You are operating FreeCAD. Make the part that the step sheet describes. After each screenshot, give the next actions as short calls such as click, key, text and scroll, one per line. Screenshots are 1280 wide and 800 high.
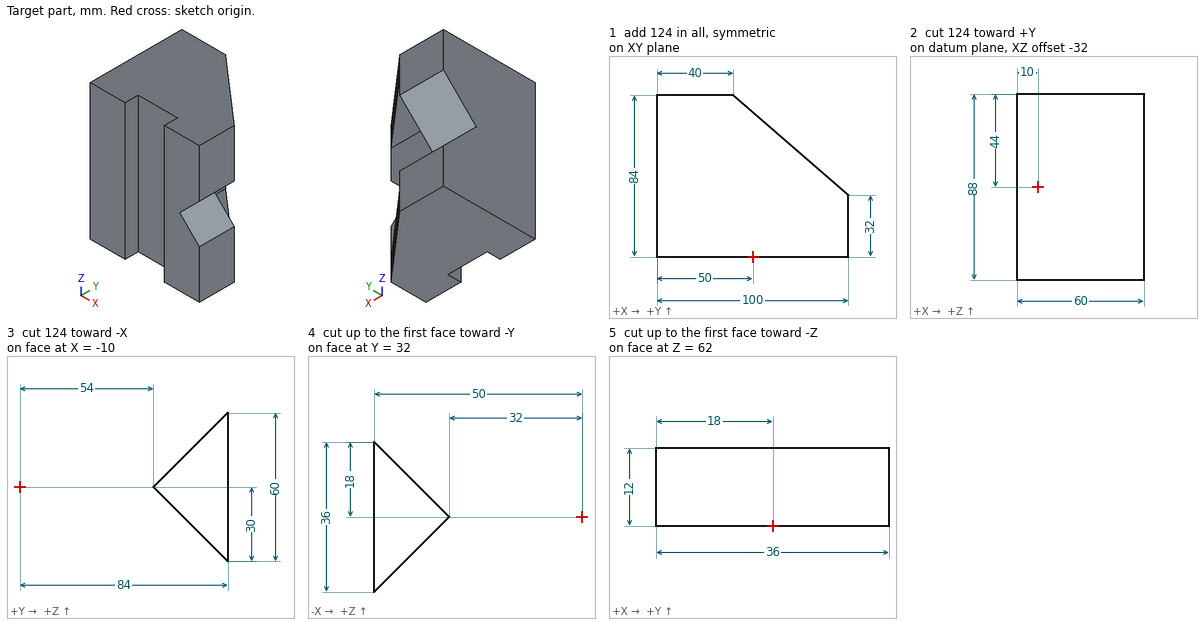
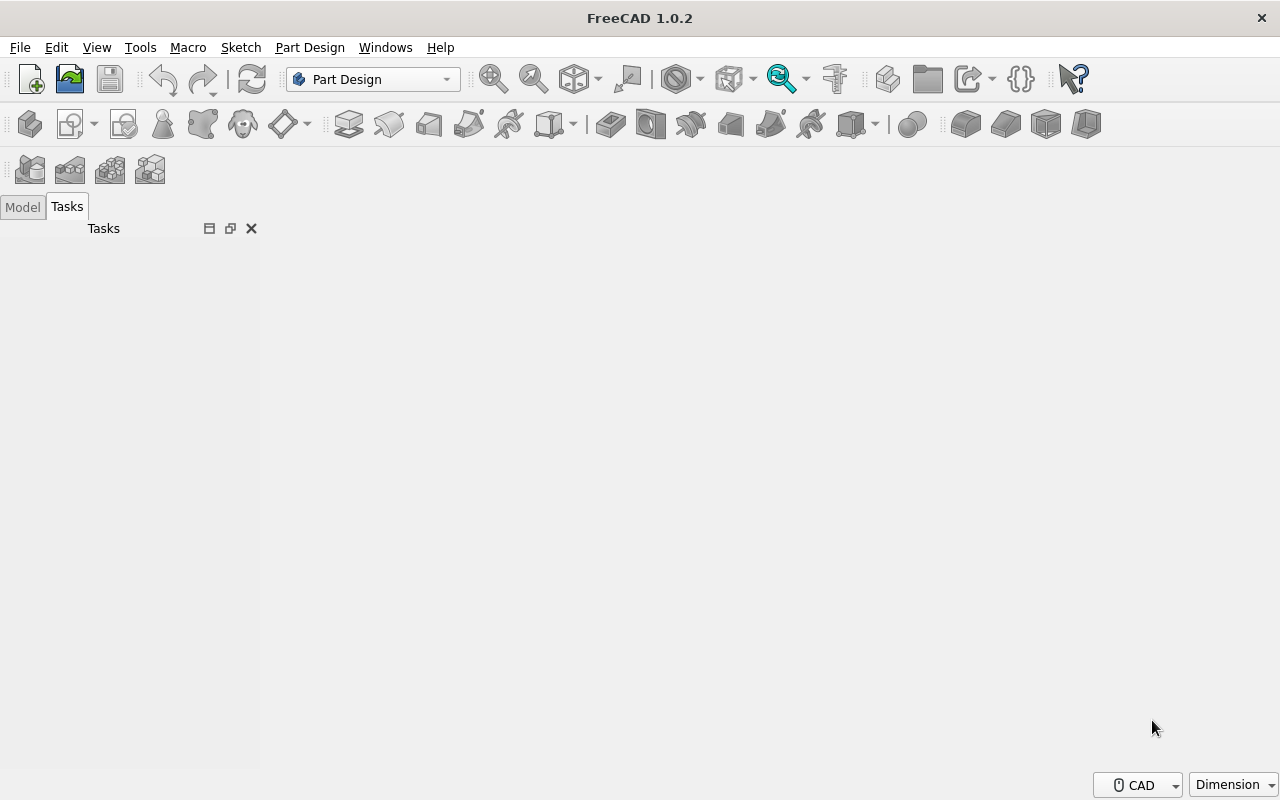
click(30, 80)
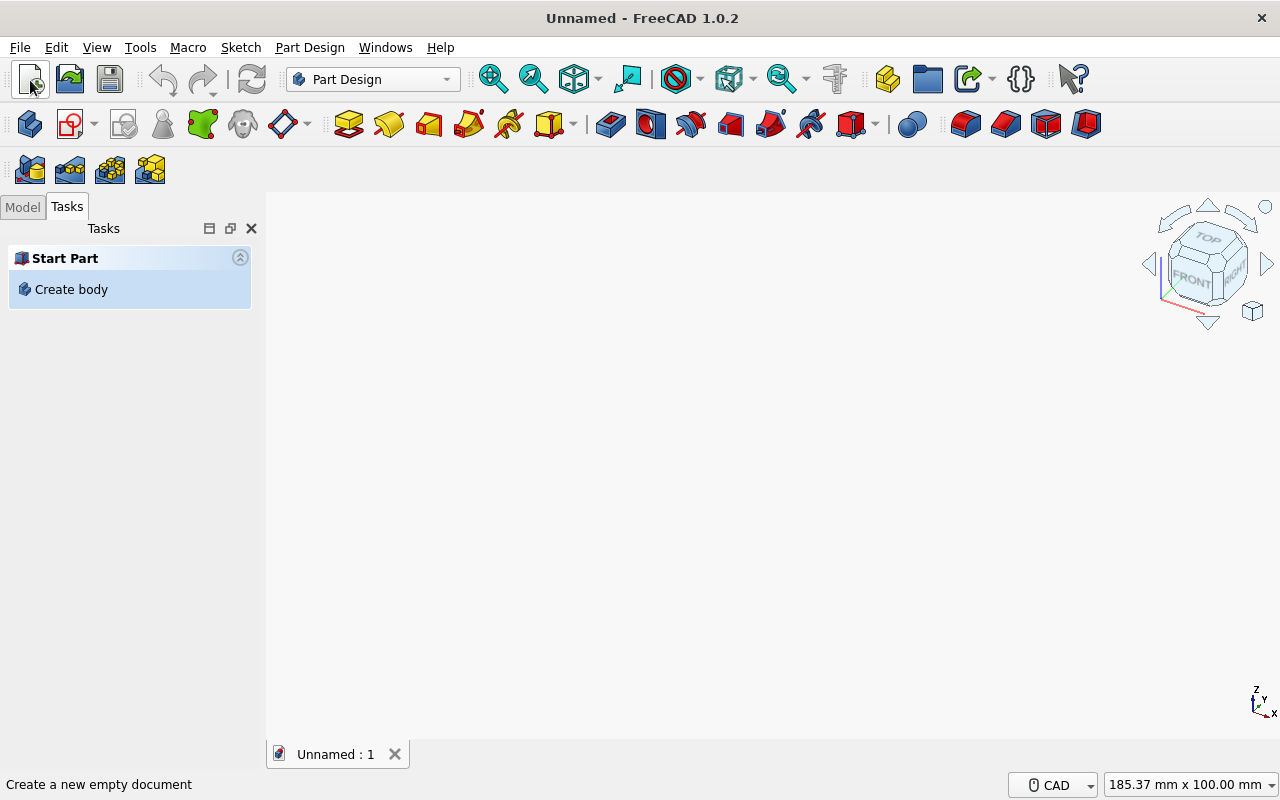
click(70, 124)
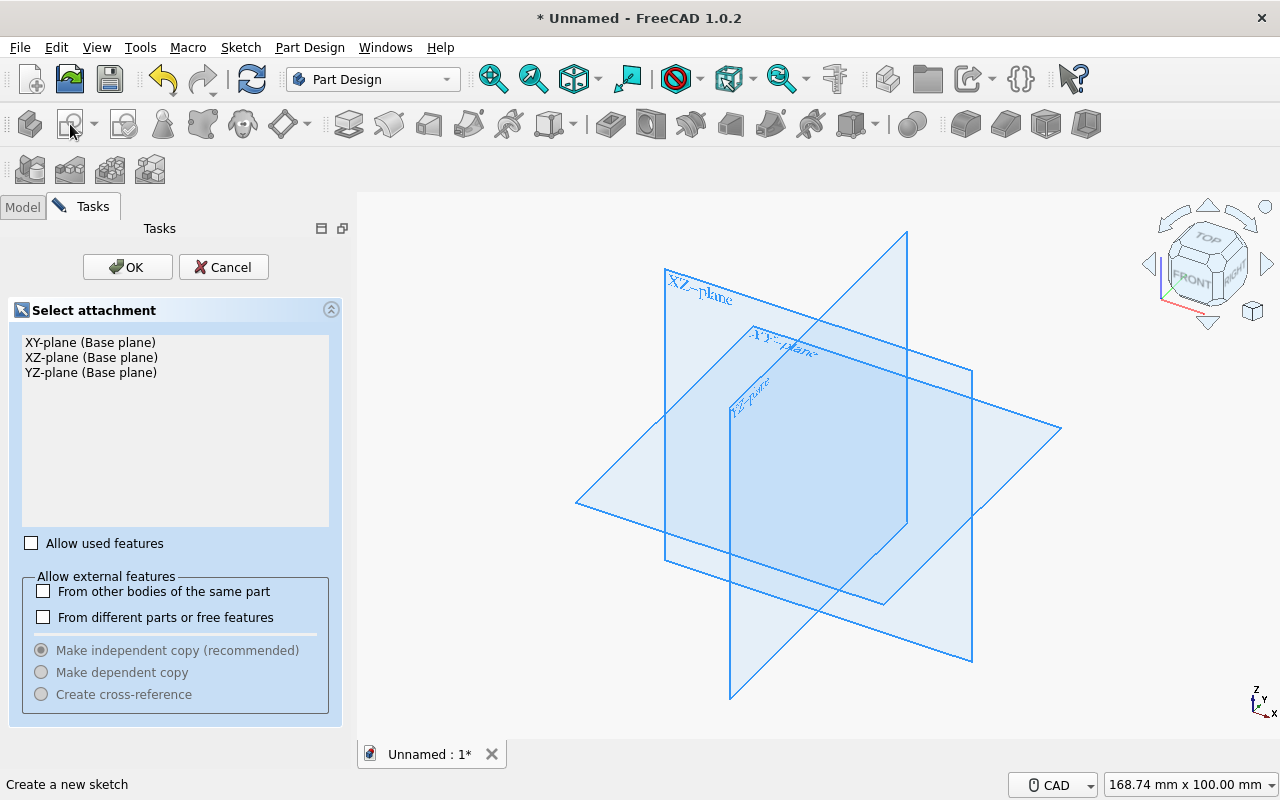
click(82, 342)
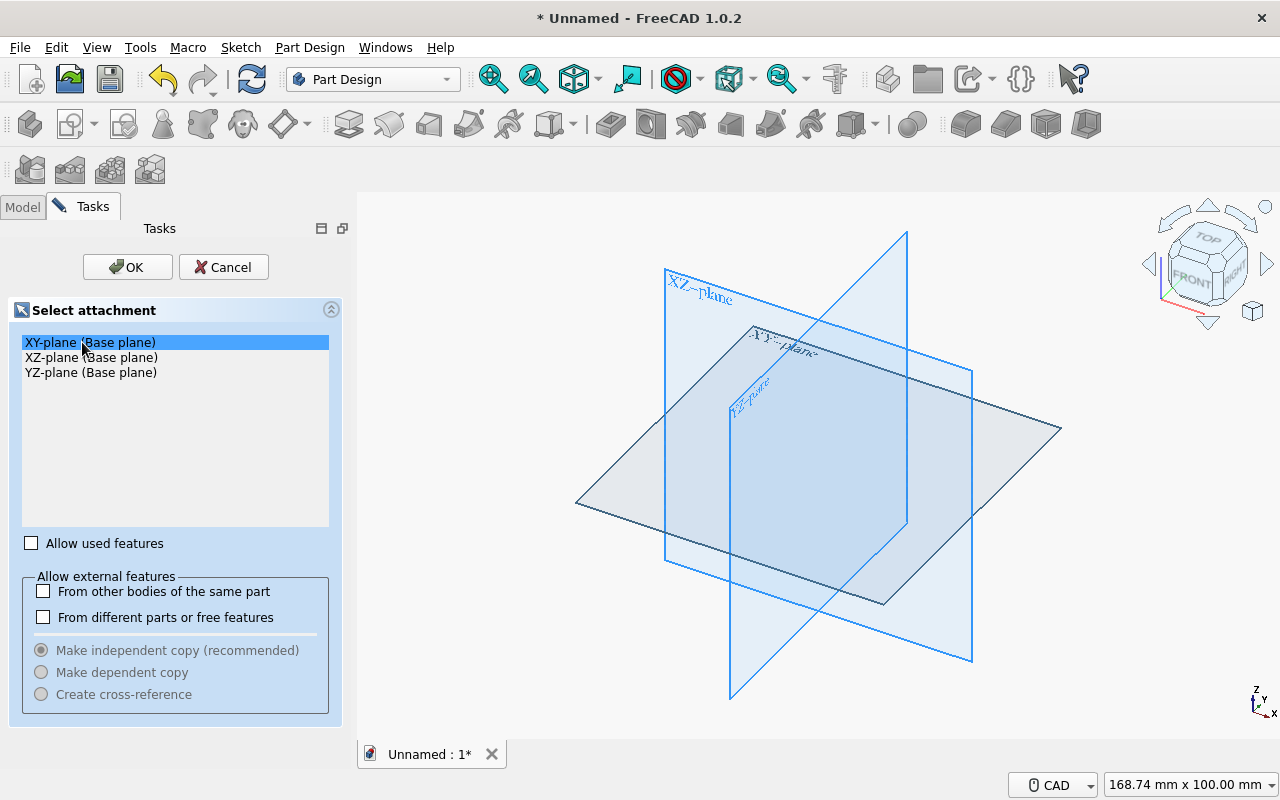
click(128, 267)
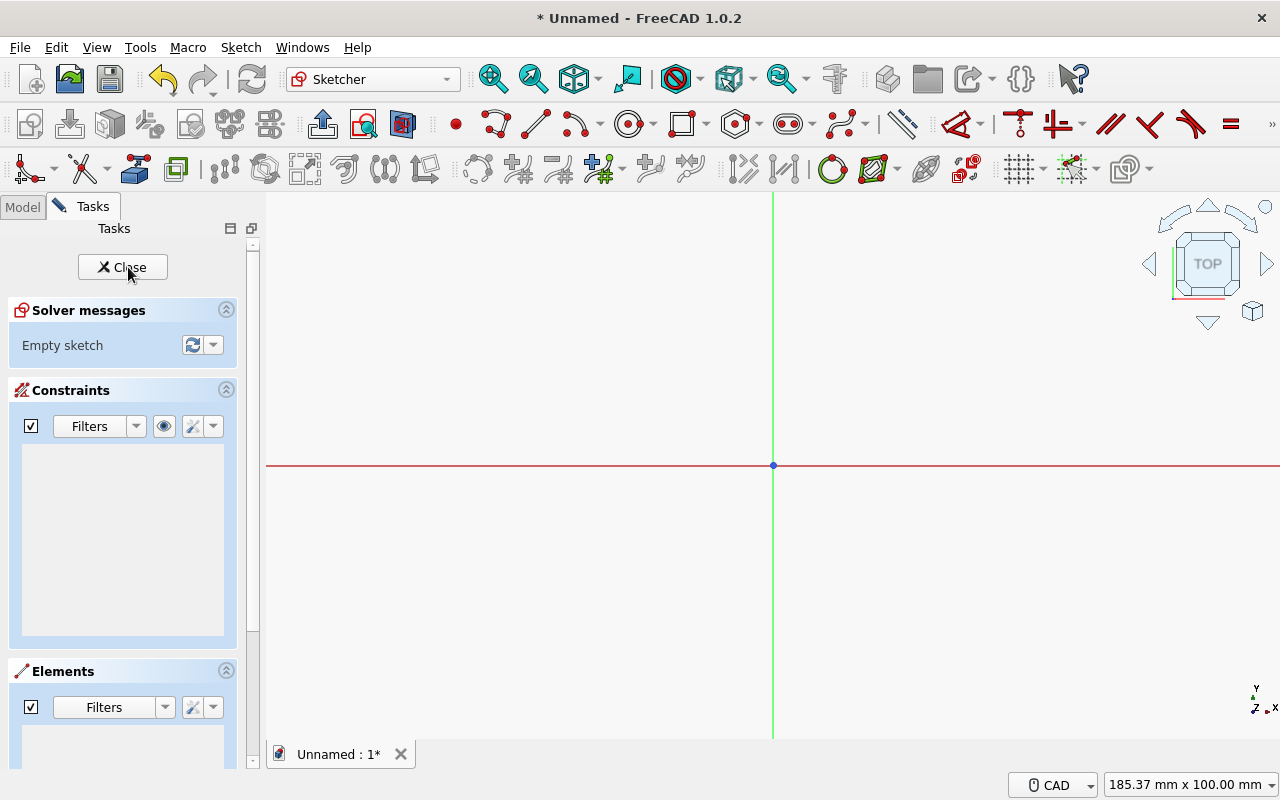
scroll(621, 711, down, 3)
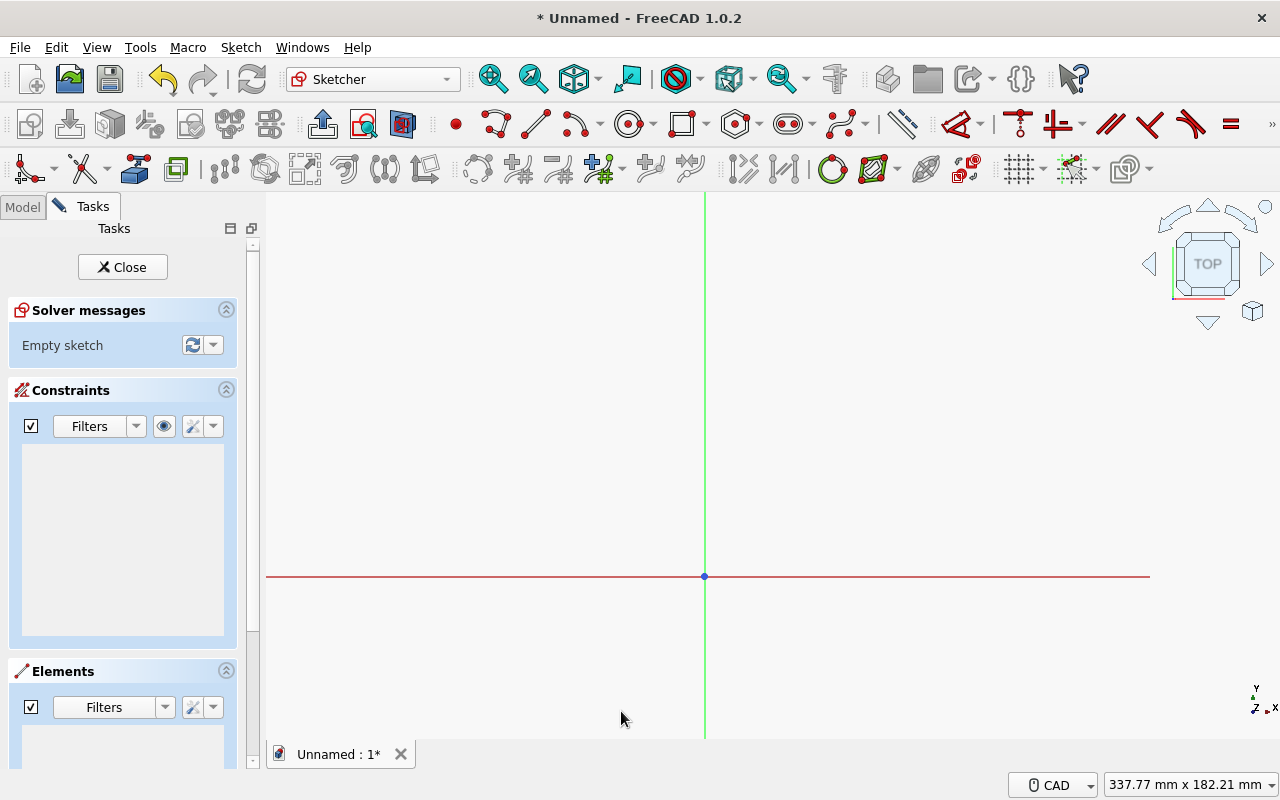
scroll(705, 420, up, 2)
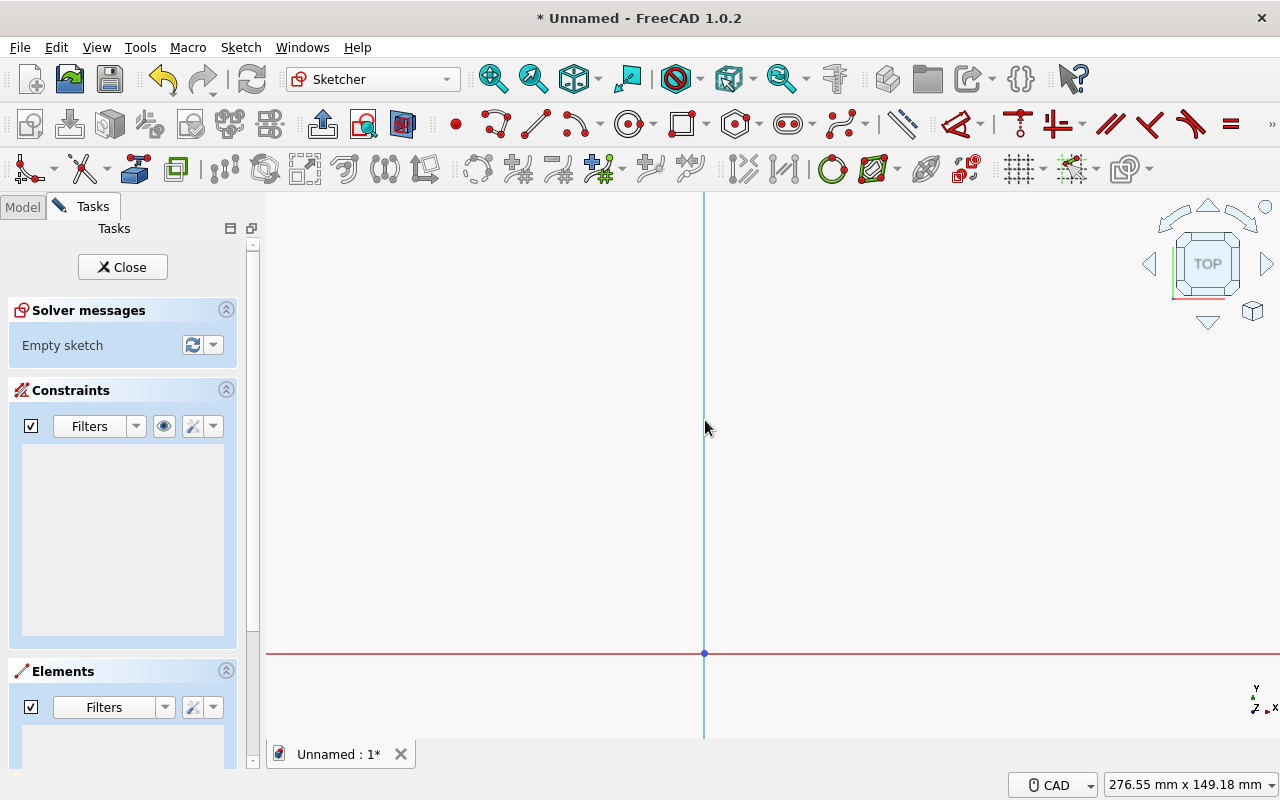
click(496, 124)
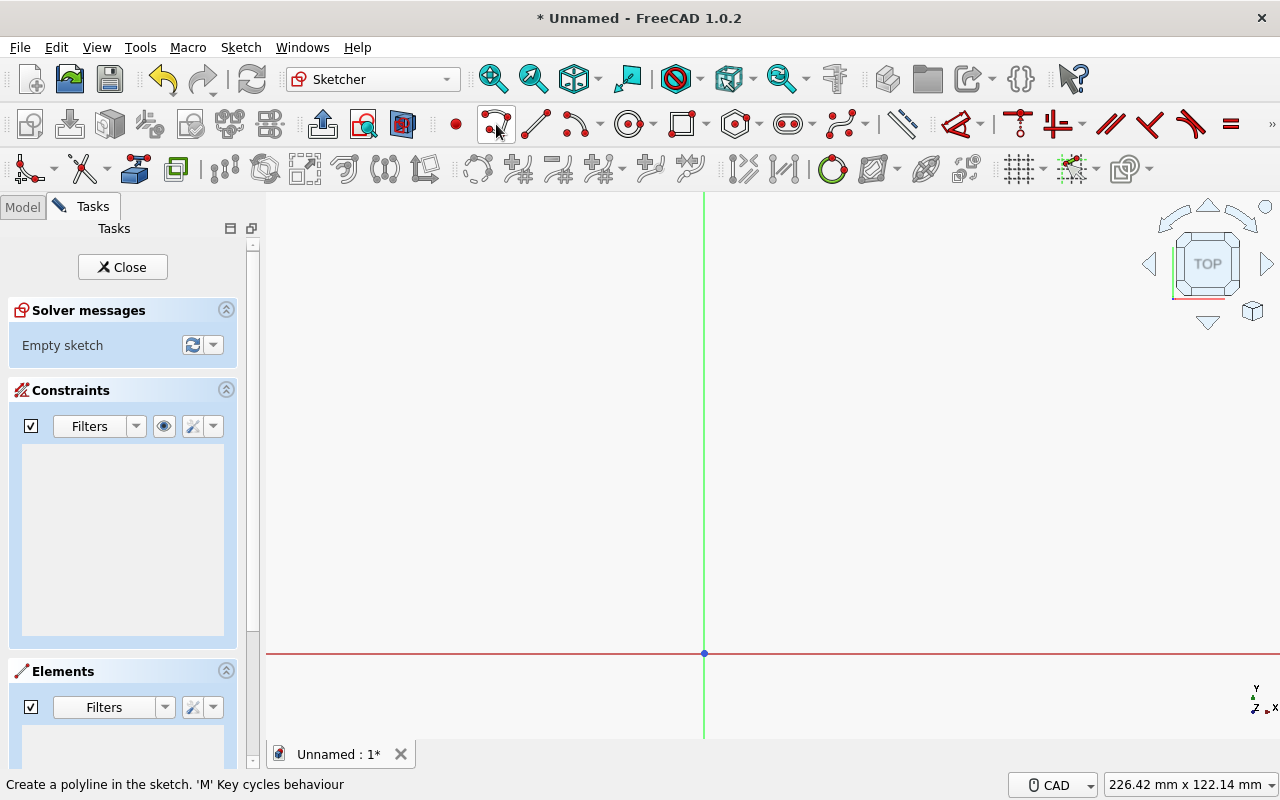
click(480, 654)
click(928, 645)
click(928, 510)
click(659, 277)
click(480, 277)
click(480, 654)
key(Escape)
key(Escape)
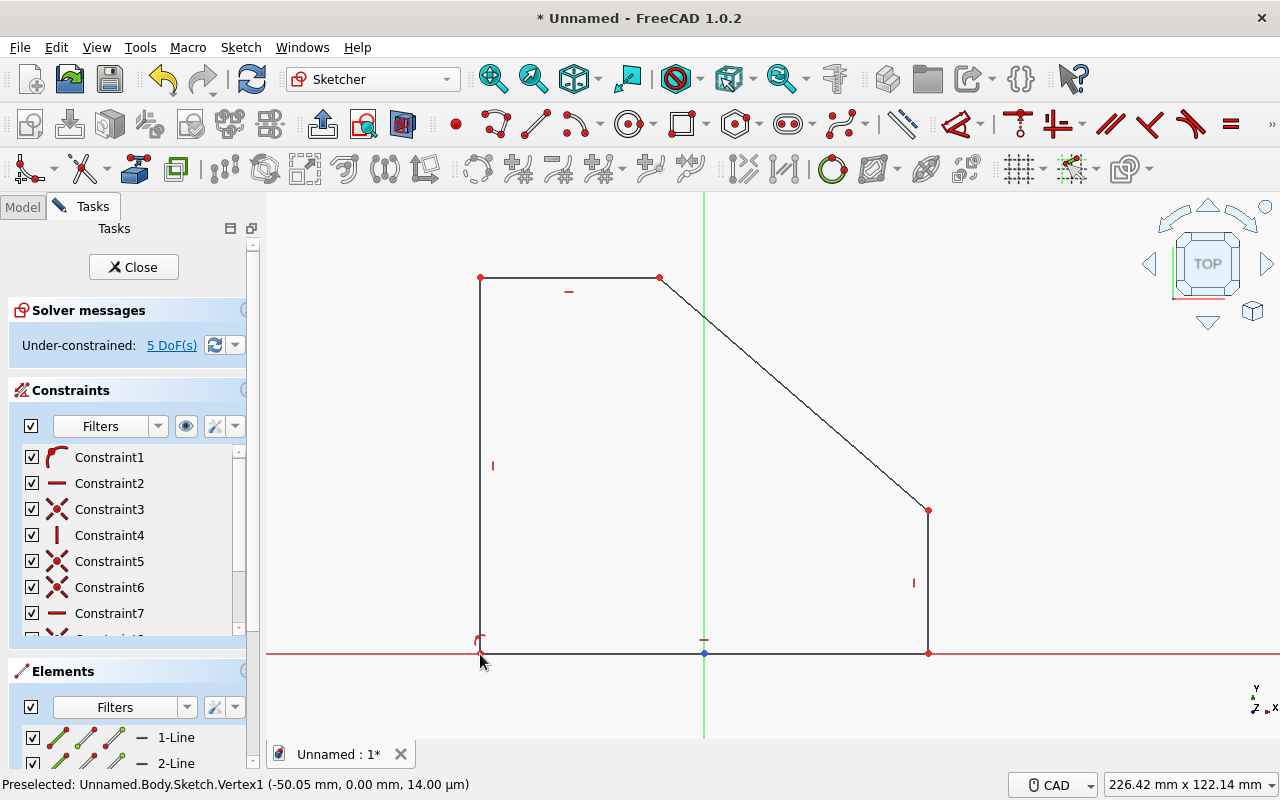
click(956, 124)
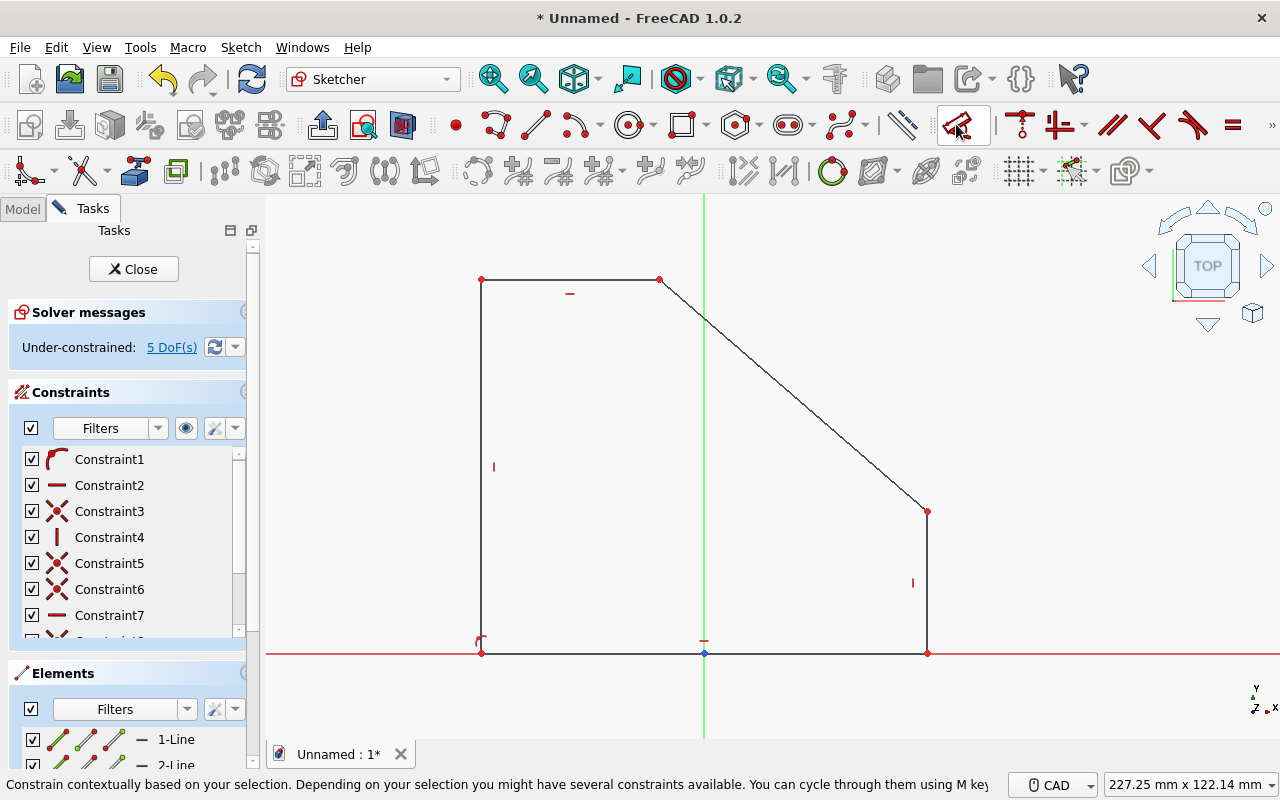
click(927, 611)
click(961, 583)